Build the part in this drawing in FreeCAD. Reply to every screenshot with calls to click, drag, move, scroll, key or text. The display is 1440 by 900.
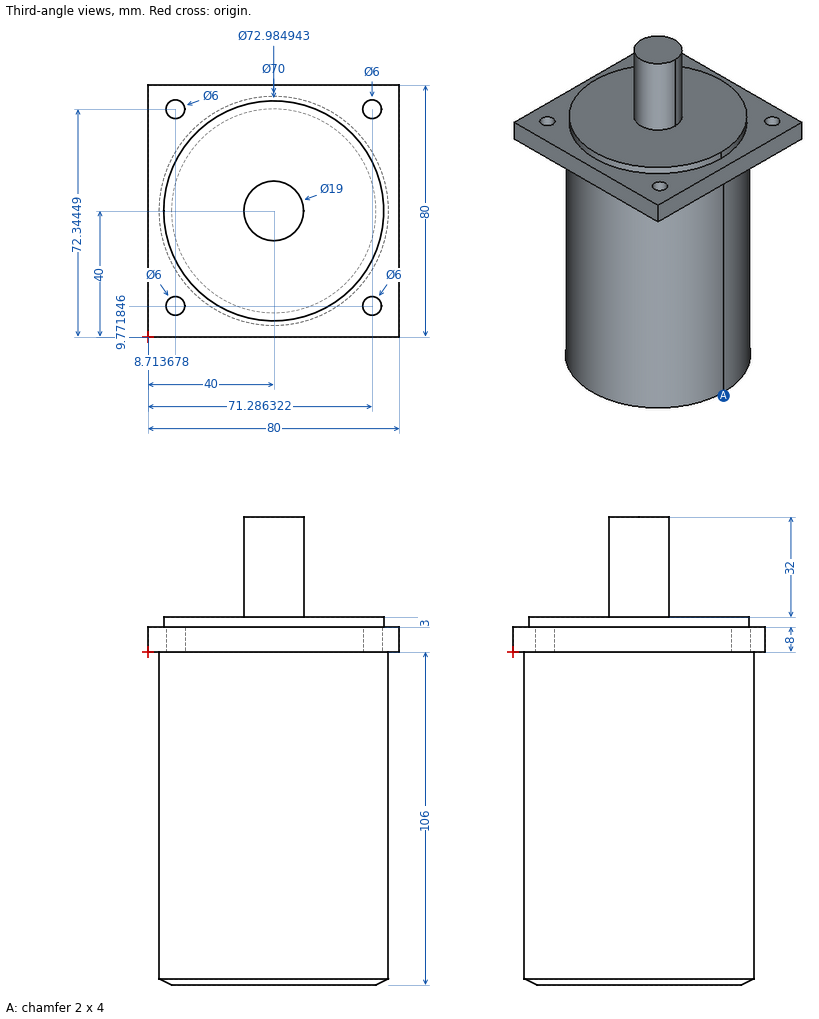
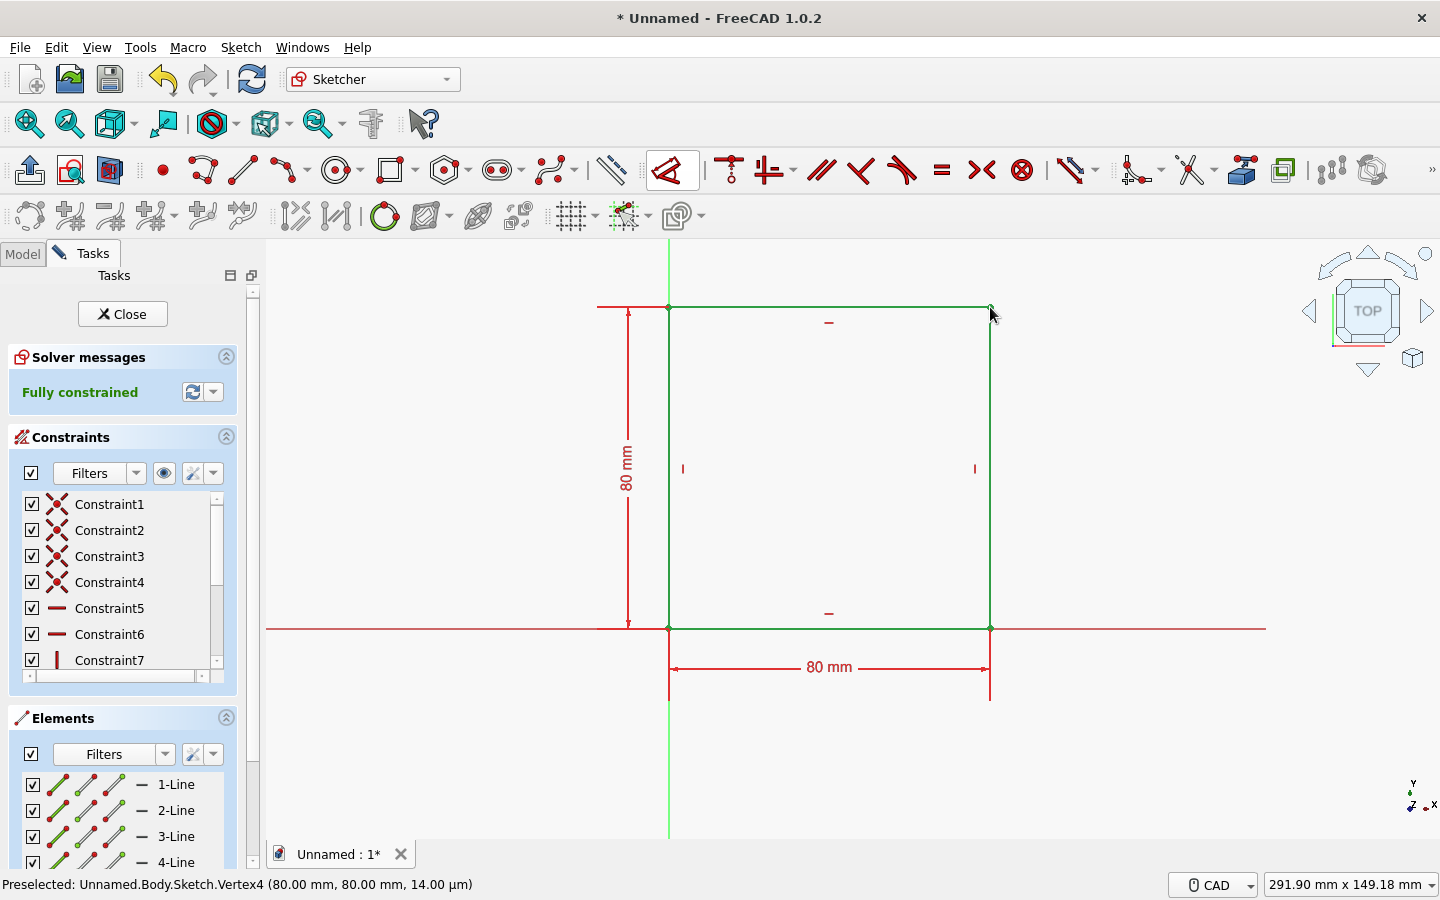
click(123, 314)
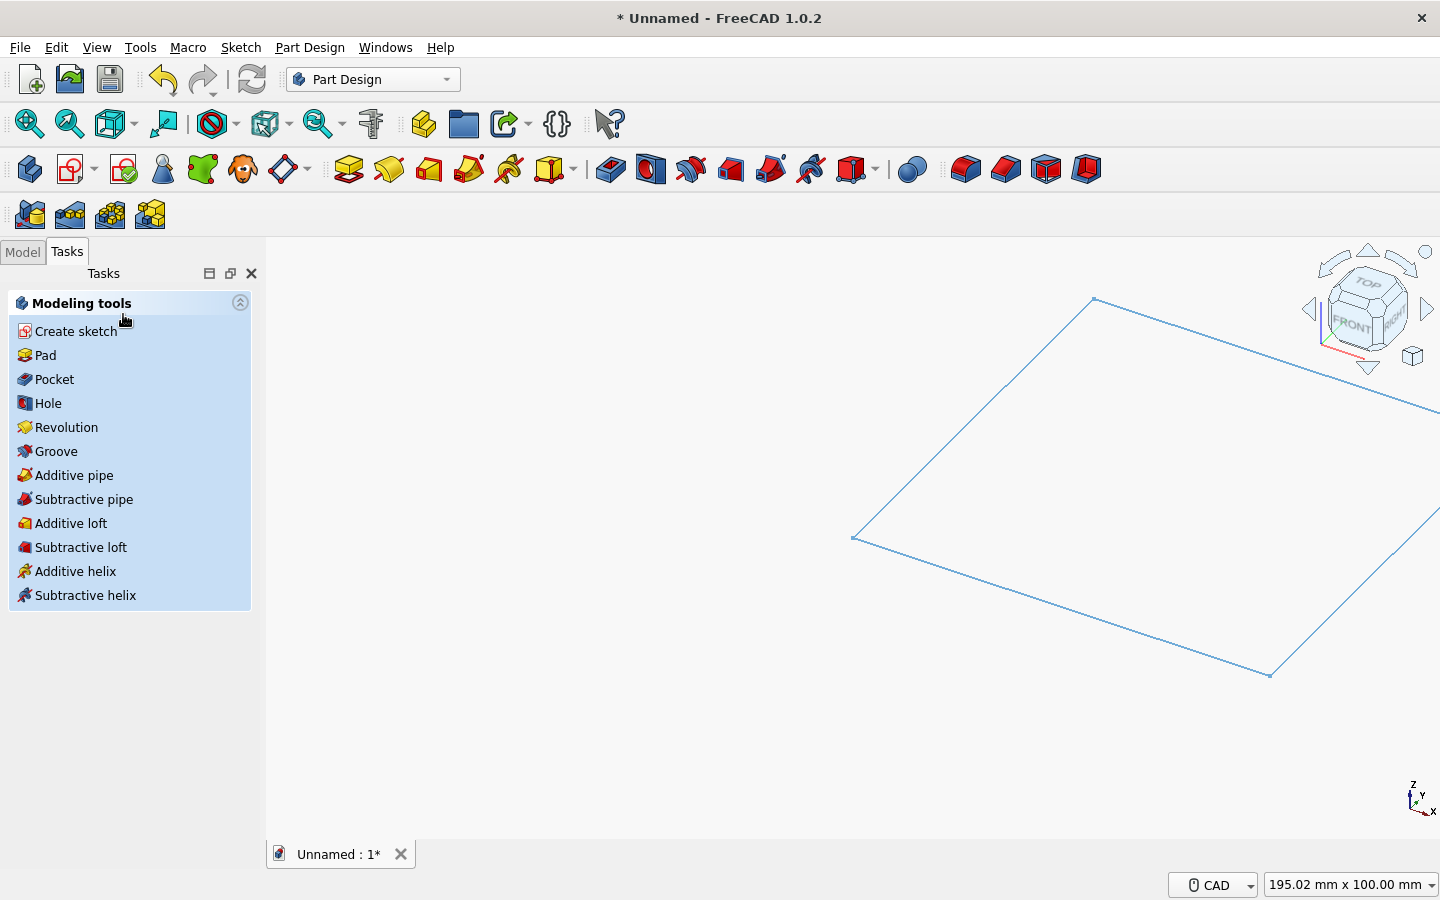
click(350, 170)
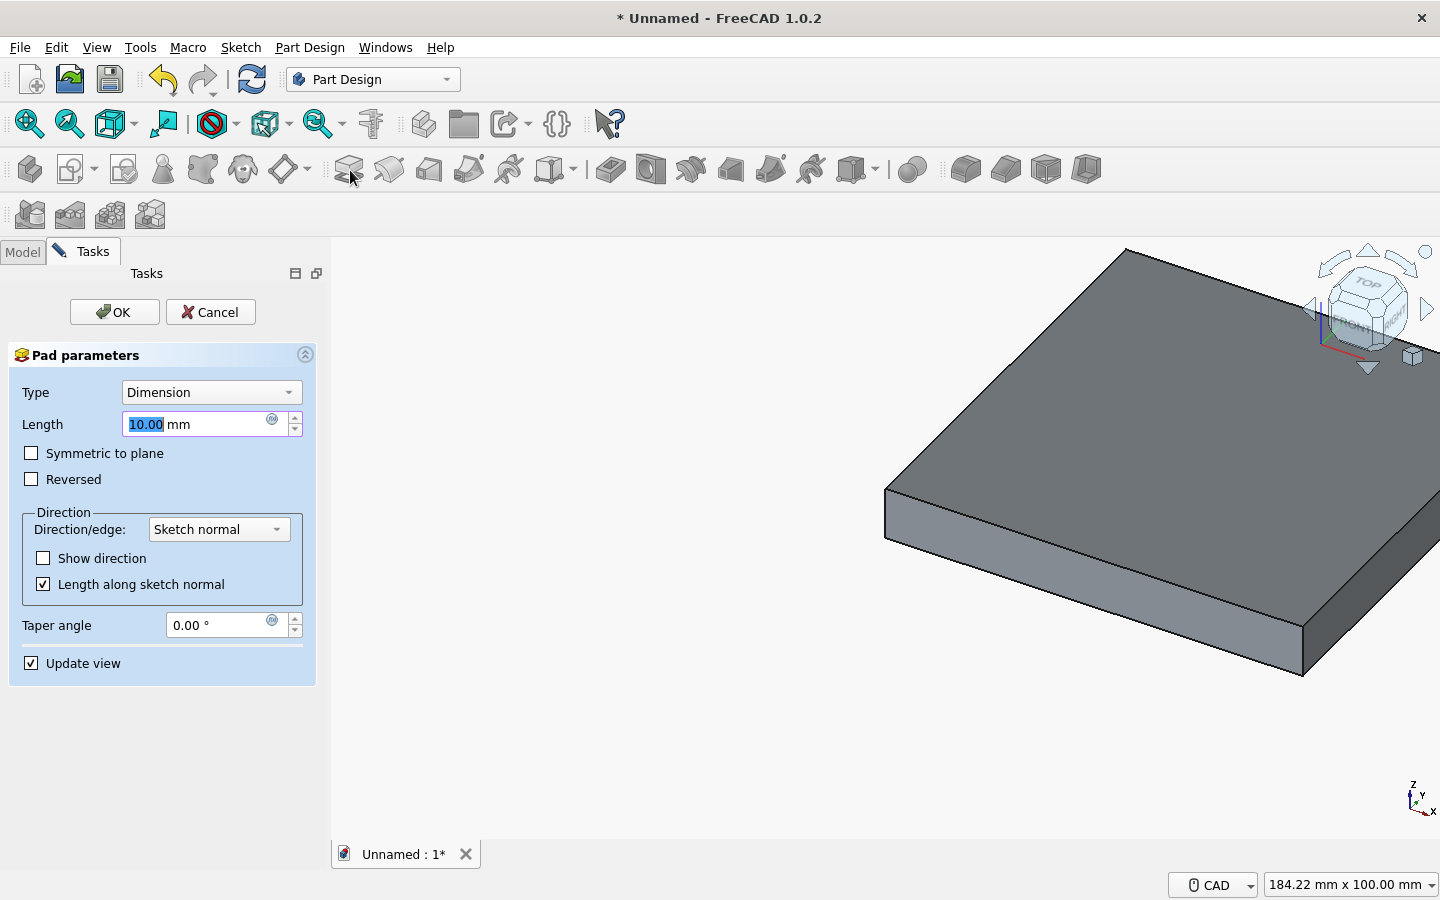
text(8)
key(Tab)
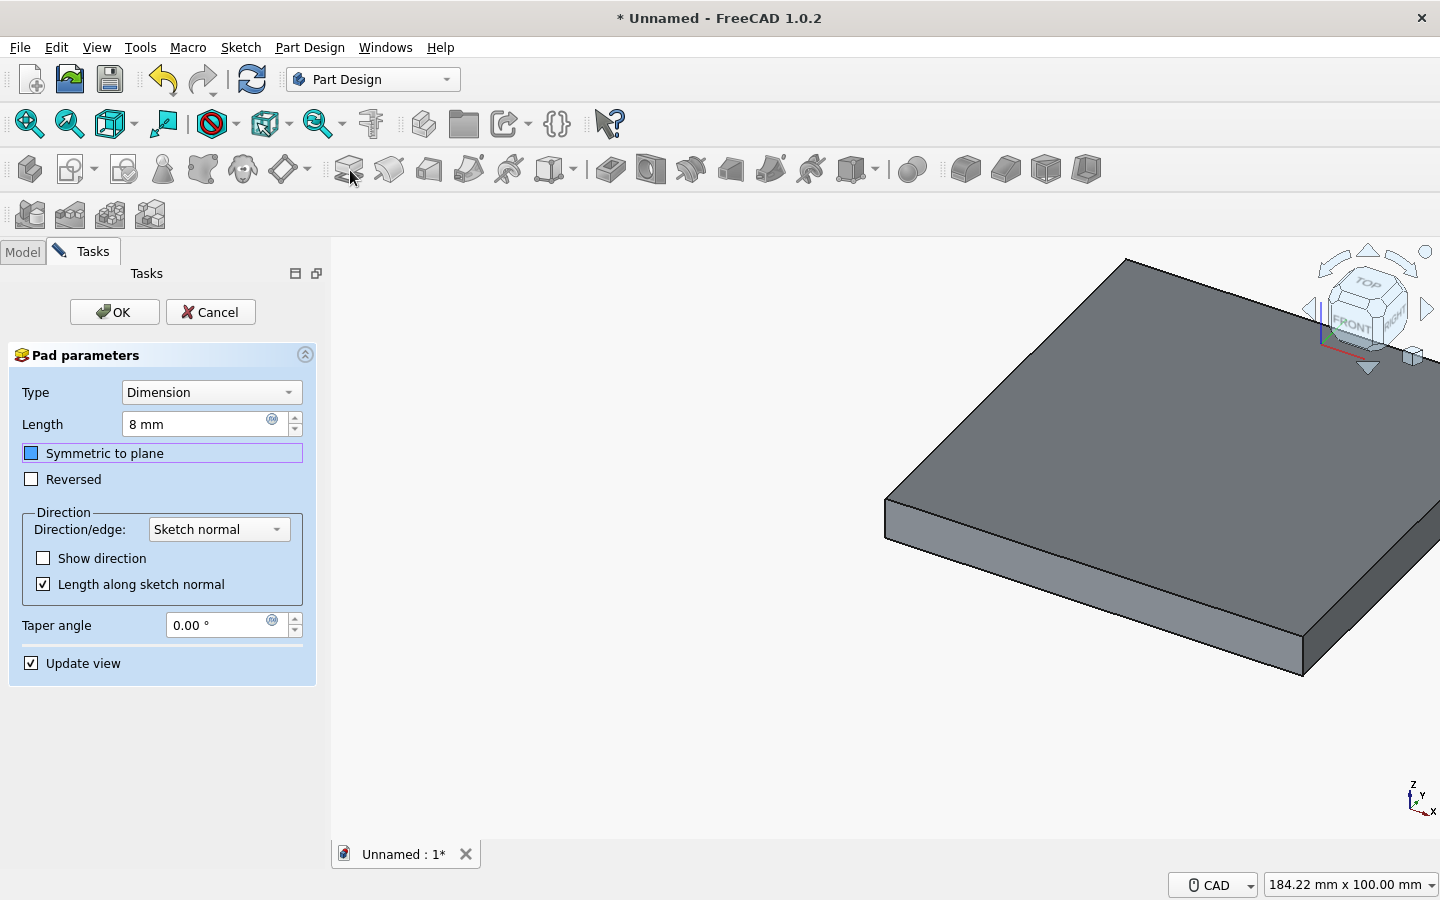
click(115, 312)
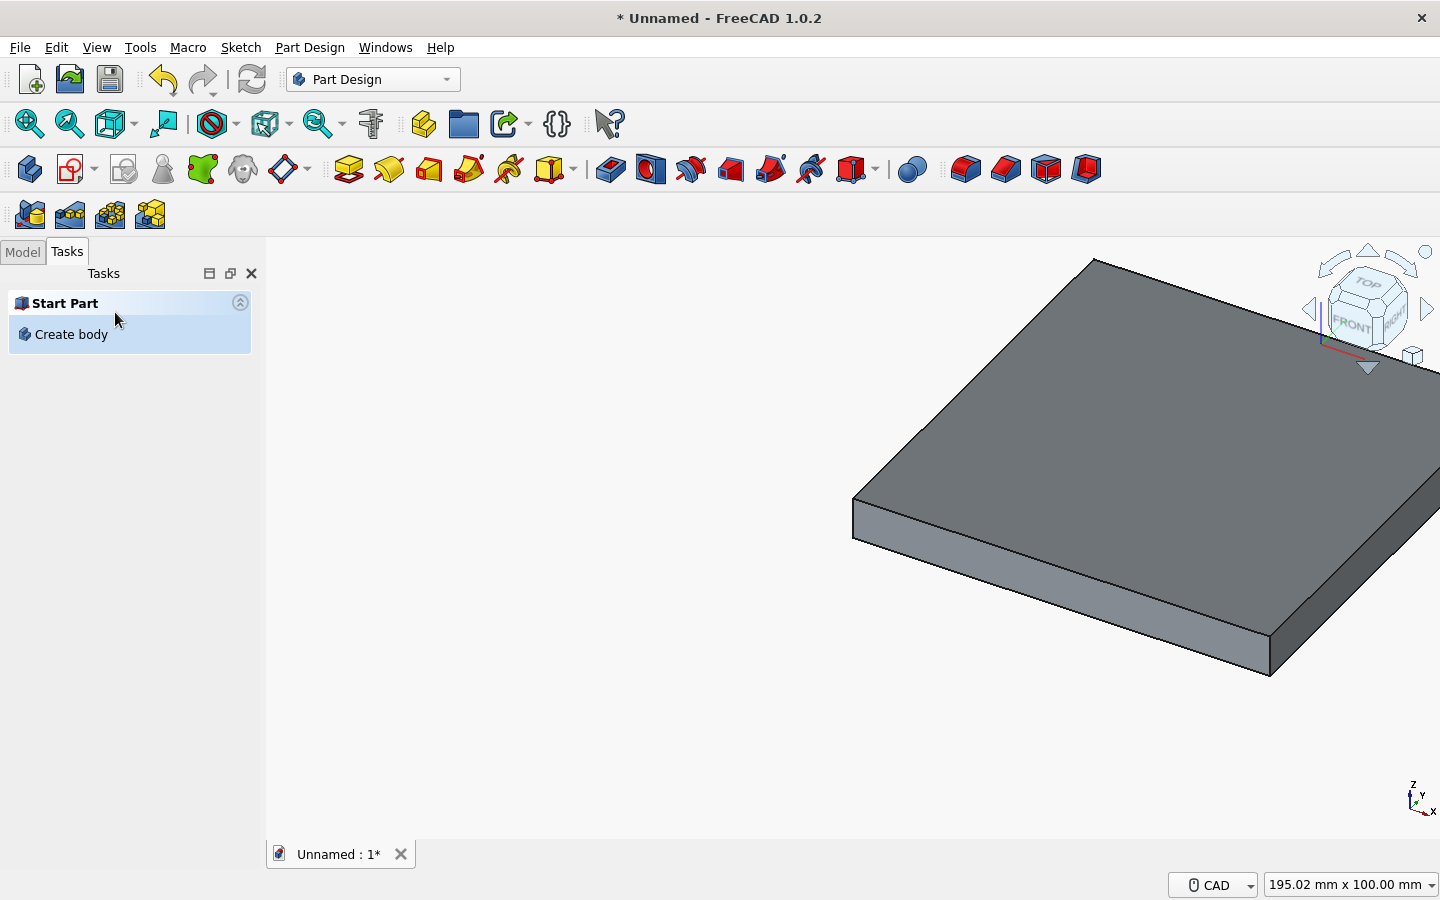
click(30, 124)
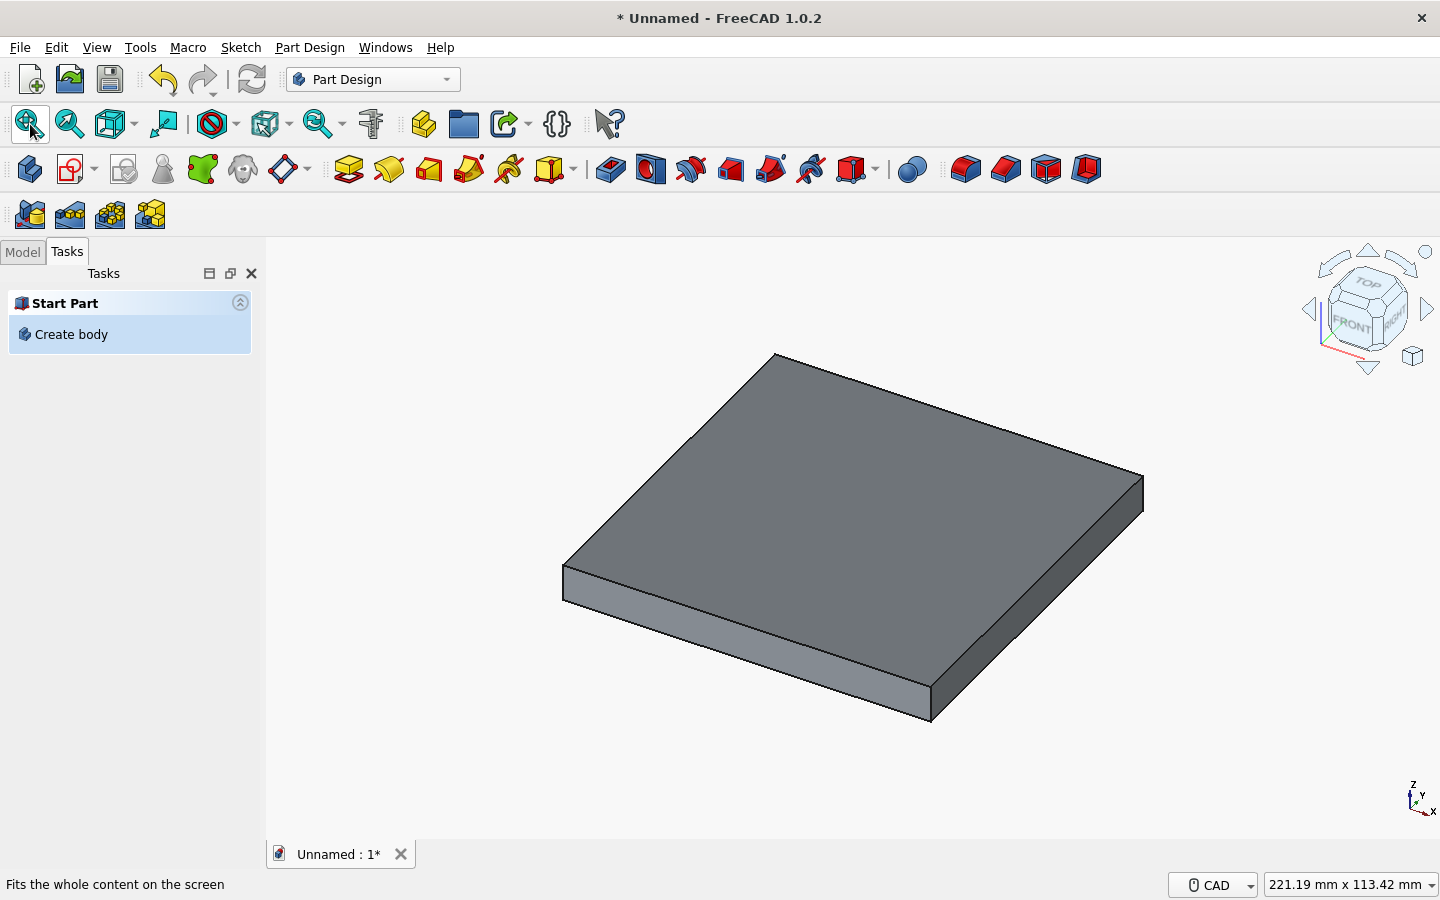
click(853, 520)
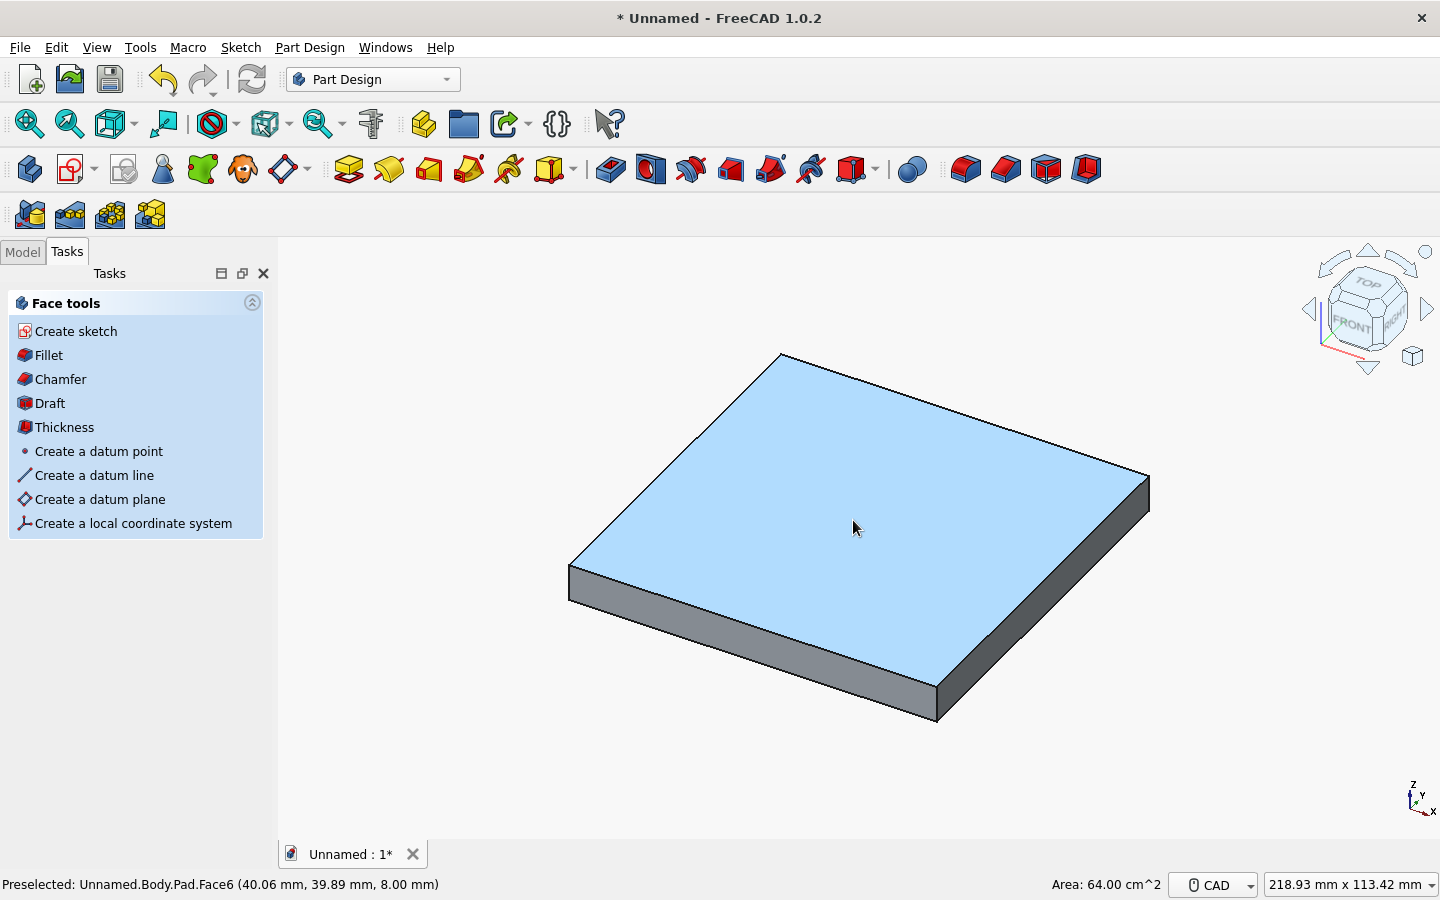
click(70, 170)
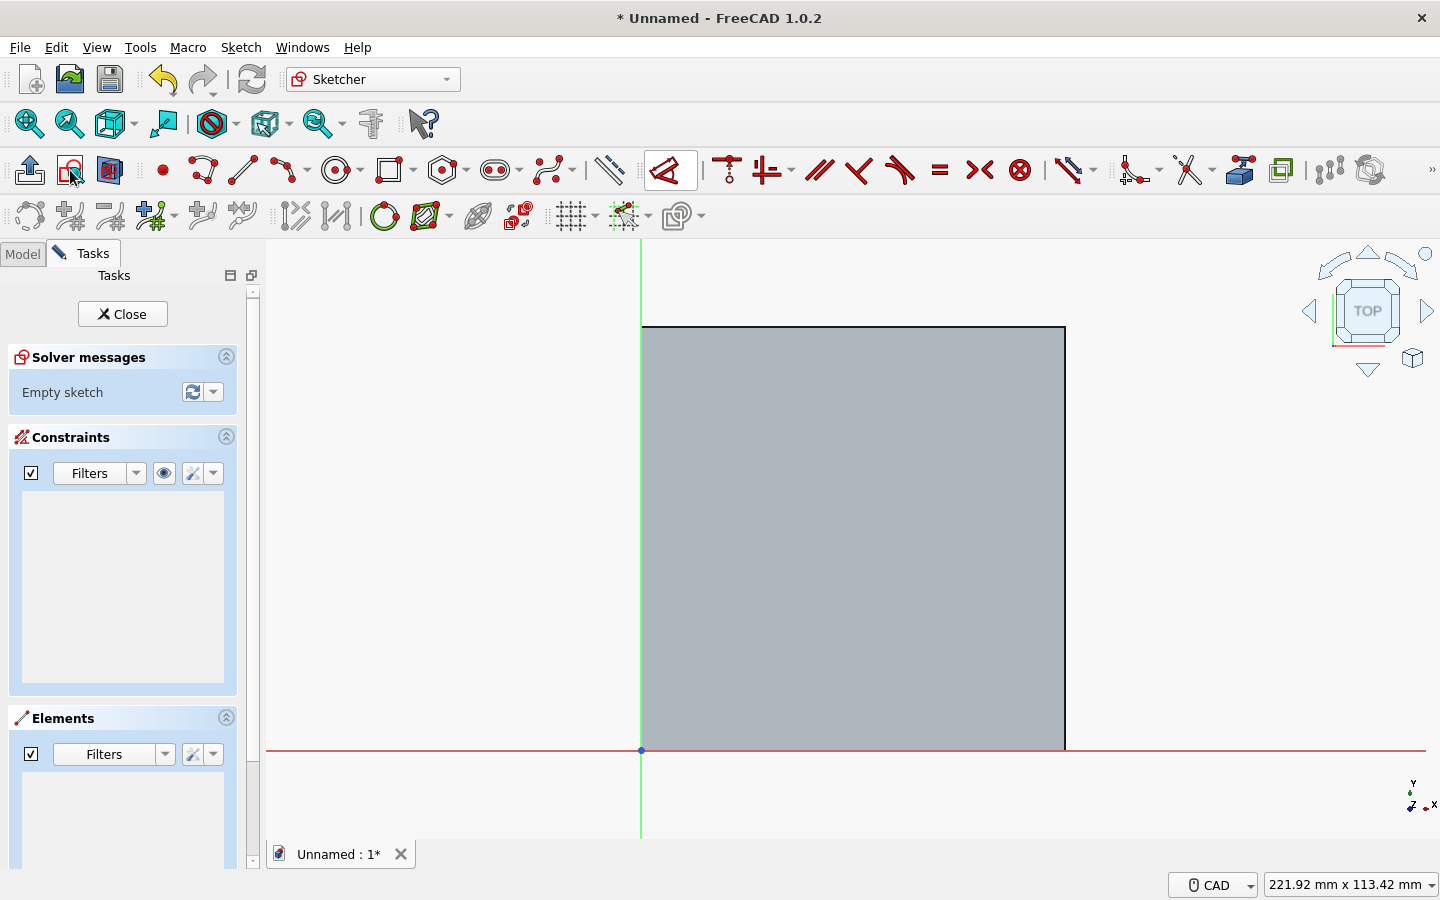
click(336, 170)